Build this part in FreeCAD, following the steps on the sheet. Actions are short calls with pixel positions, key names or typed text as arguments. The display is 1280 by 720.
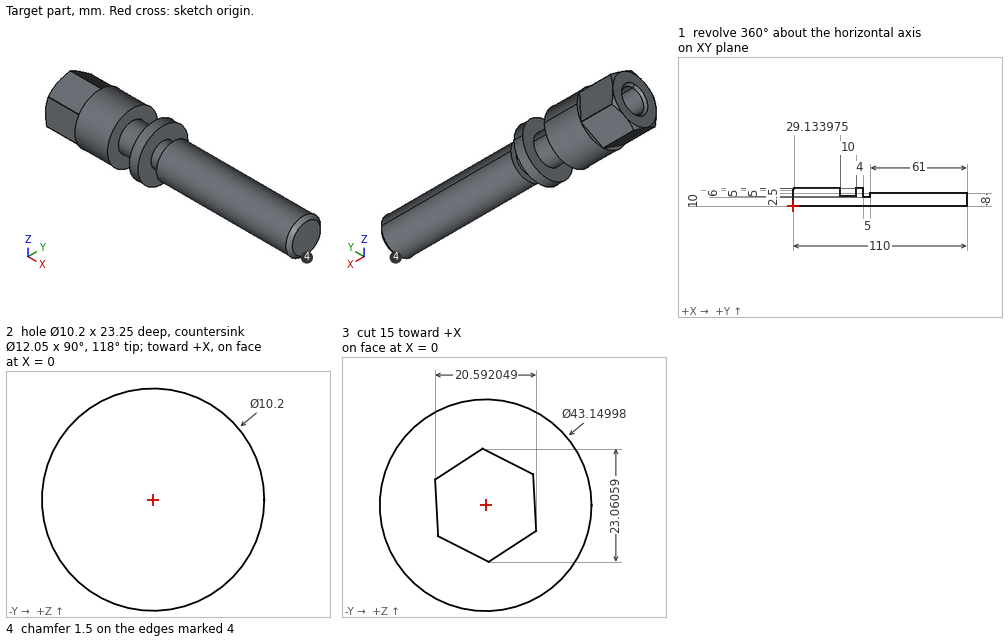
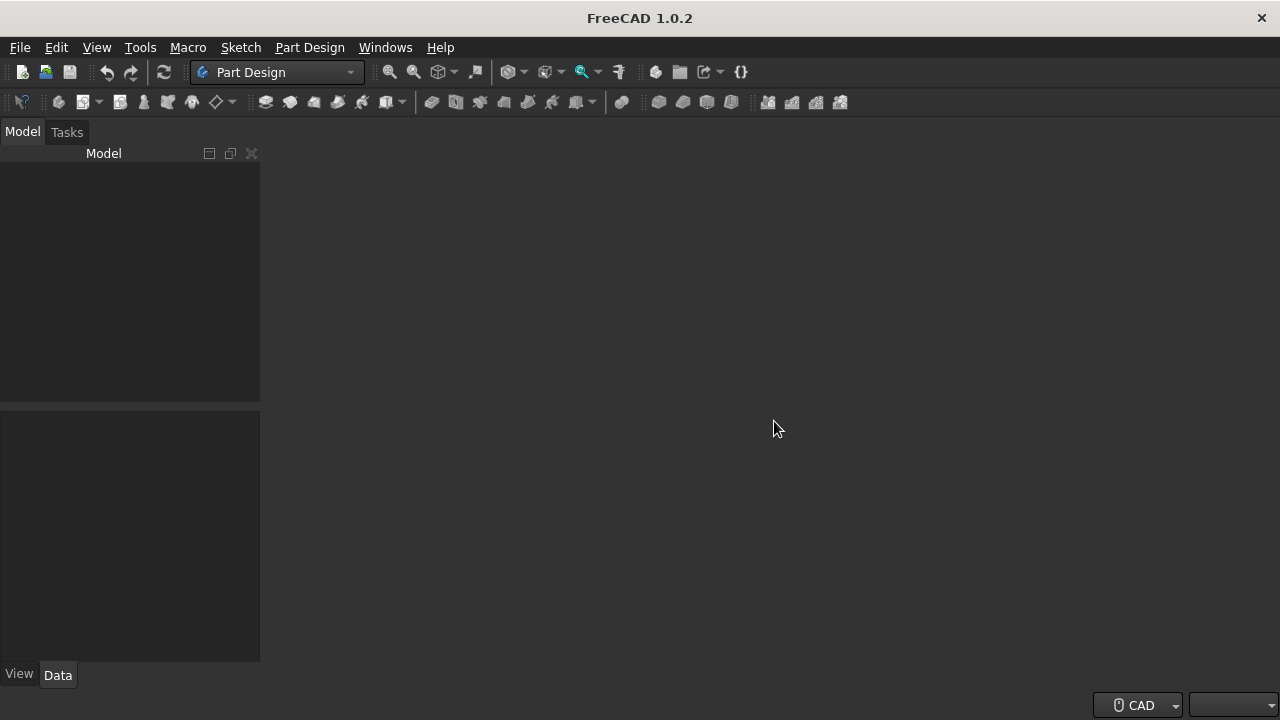
key(ctrl+n)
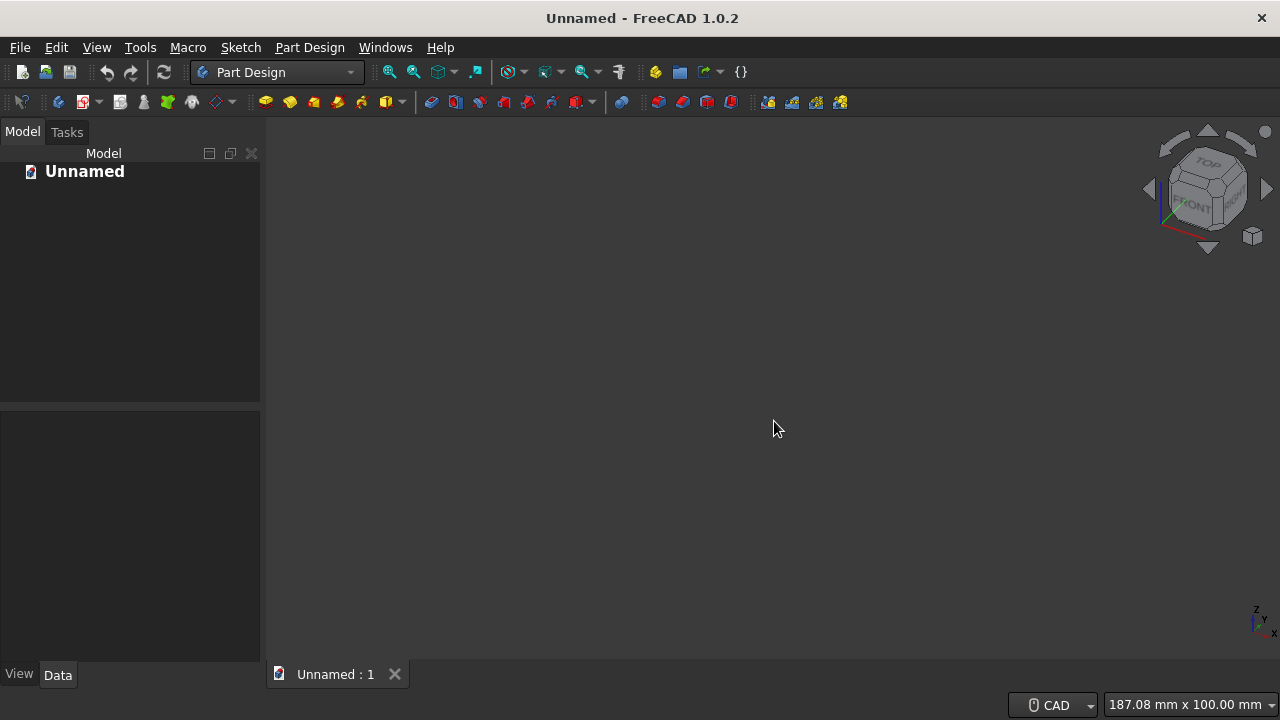
click(84, 102)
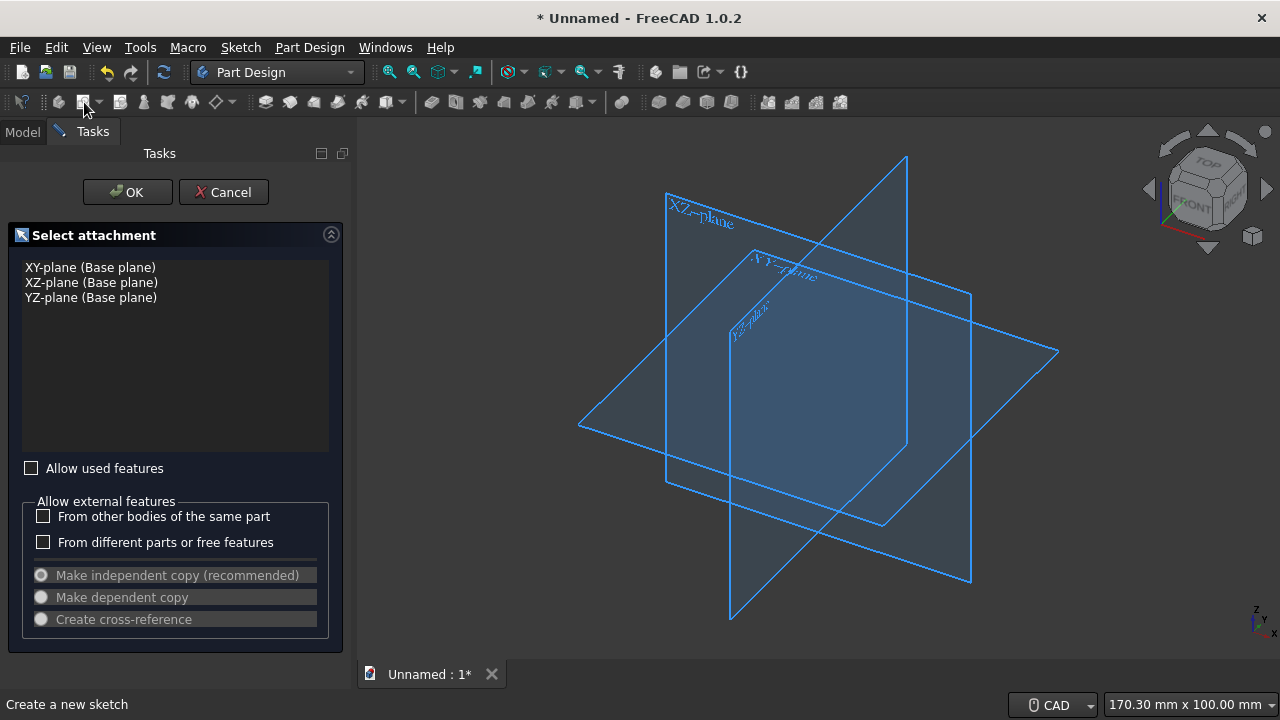
click(82, 268)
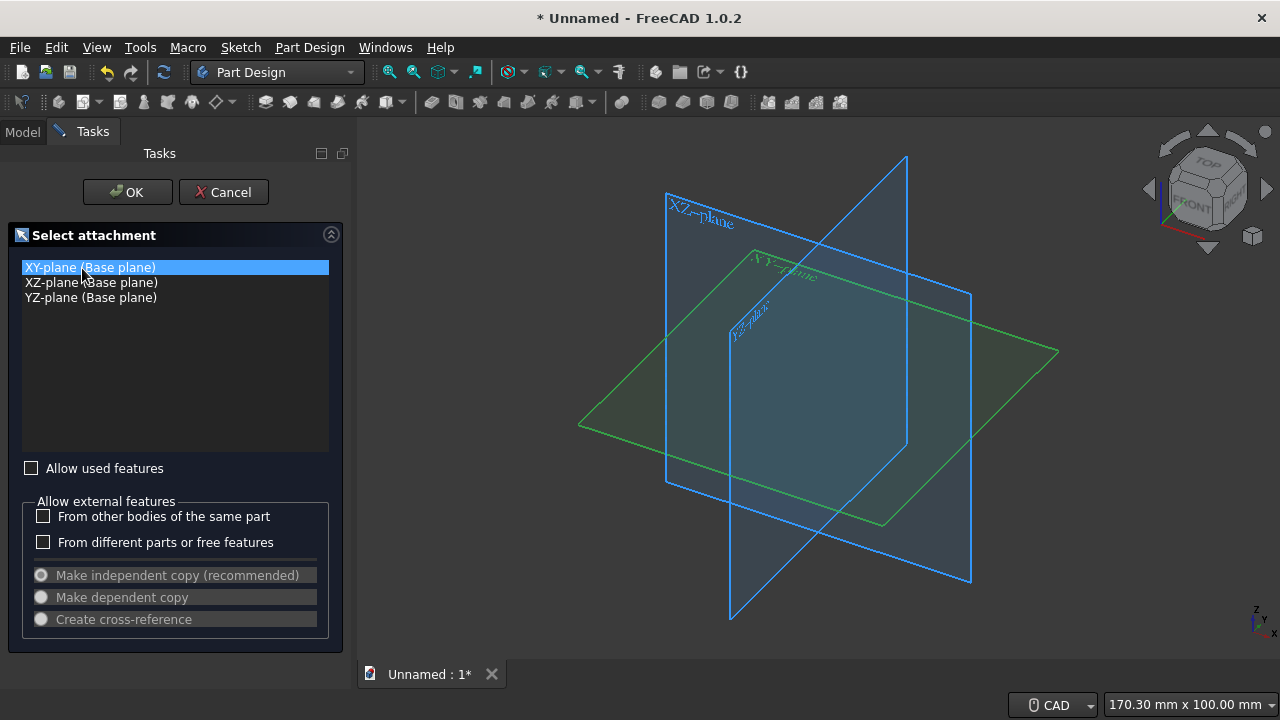
click(128, 192)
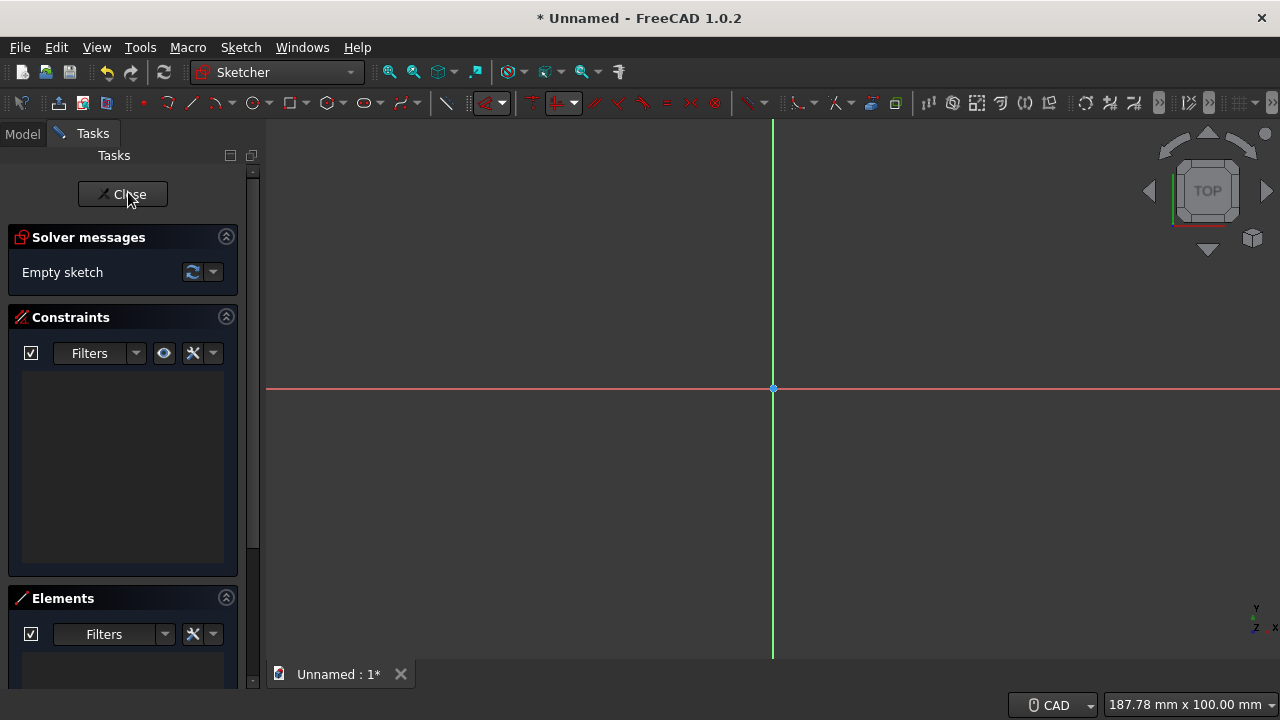
scroll(294, 452, down, 2)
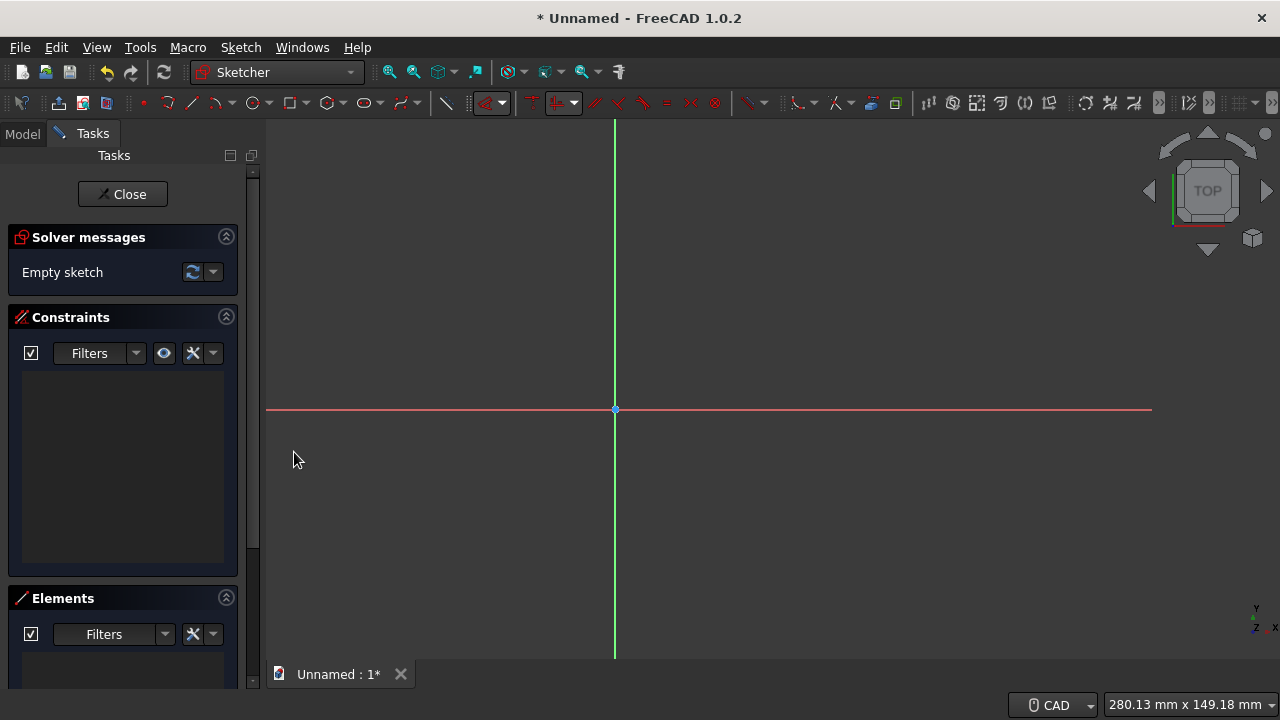
scroll(1037, 389, up, 2)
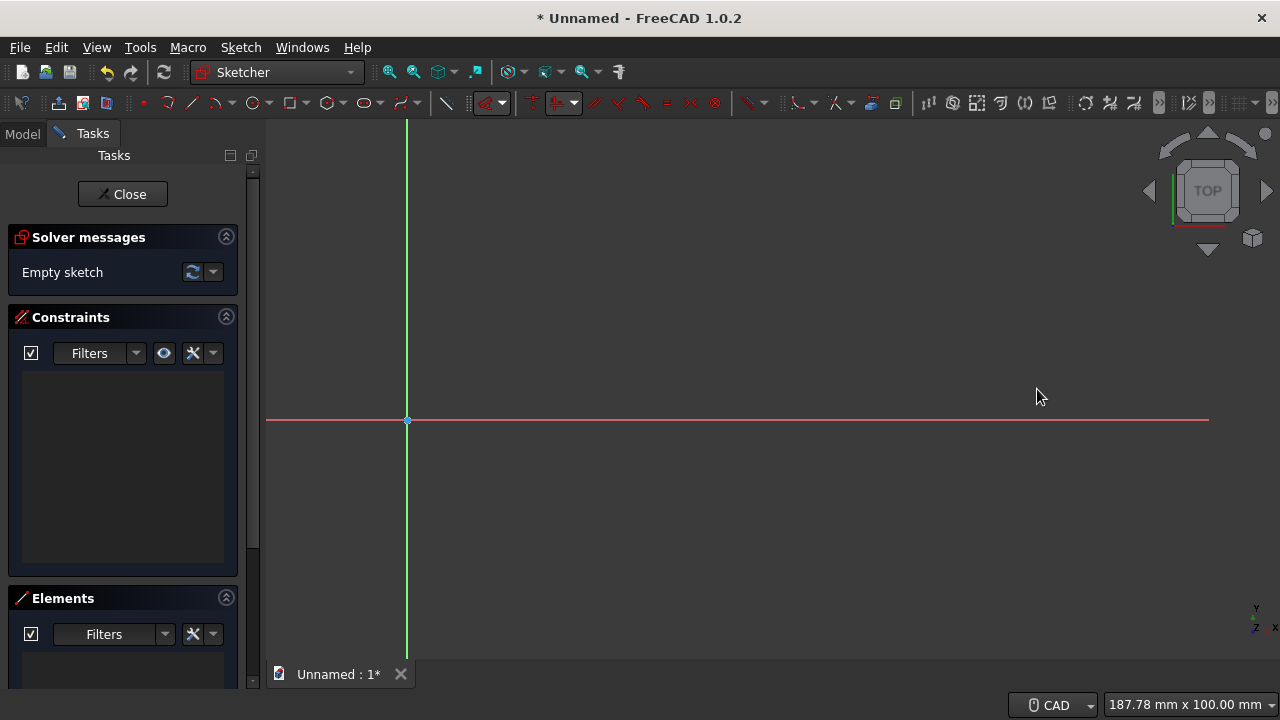
click(168, 104)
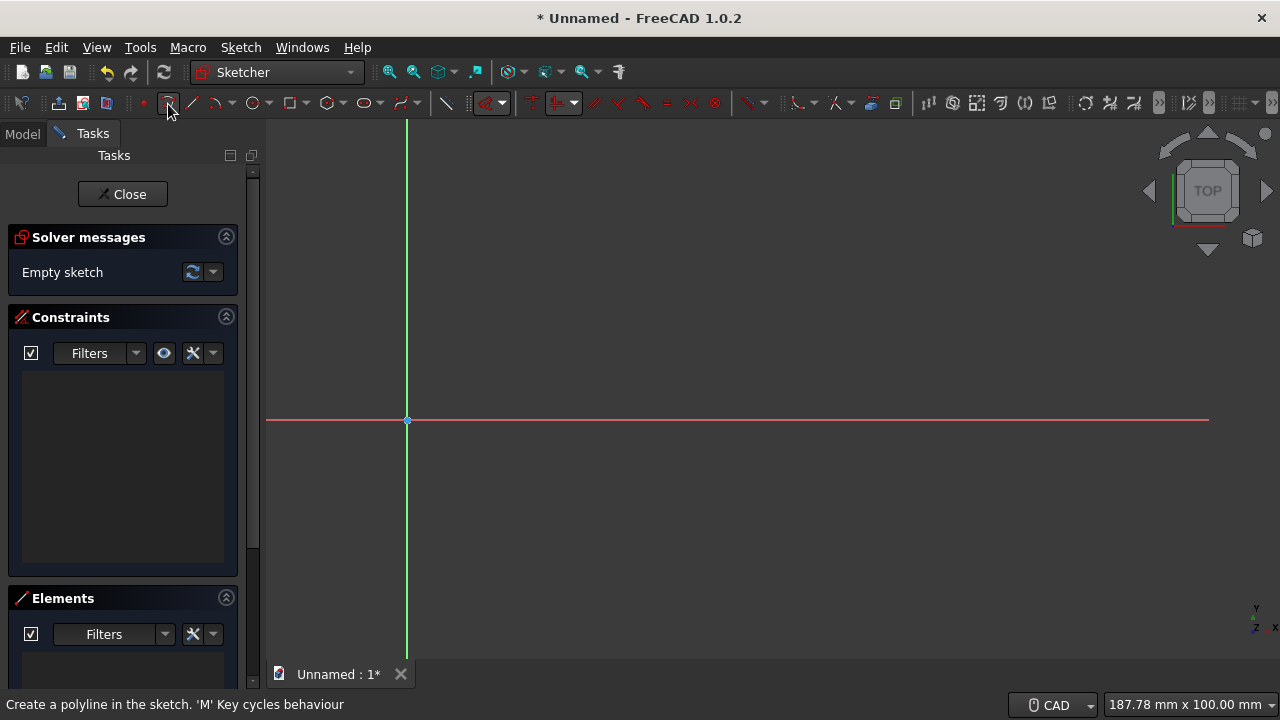
click(407, 420)
click(1001, 411)
click(1001, 377)
click(672, 377)
click(672, 390)
click(645, 390)
click(645, 358)
click(623, 358)
click(623, 385)
click(569, 385)
click(569, 358)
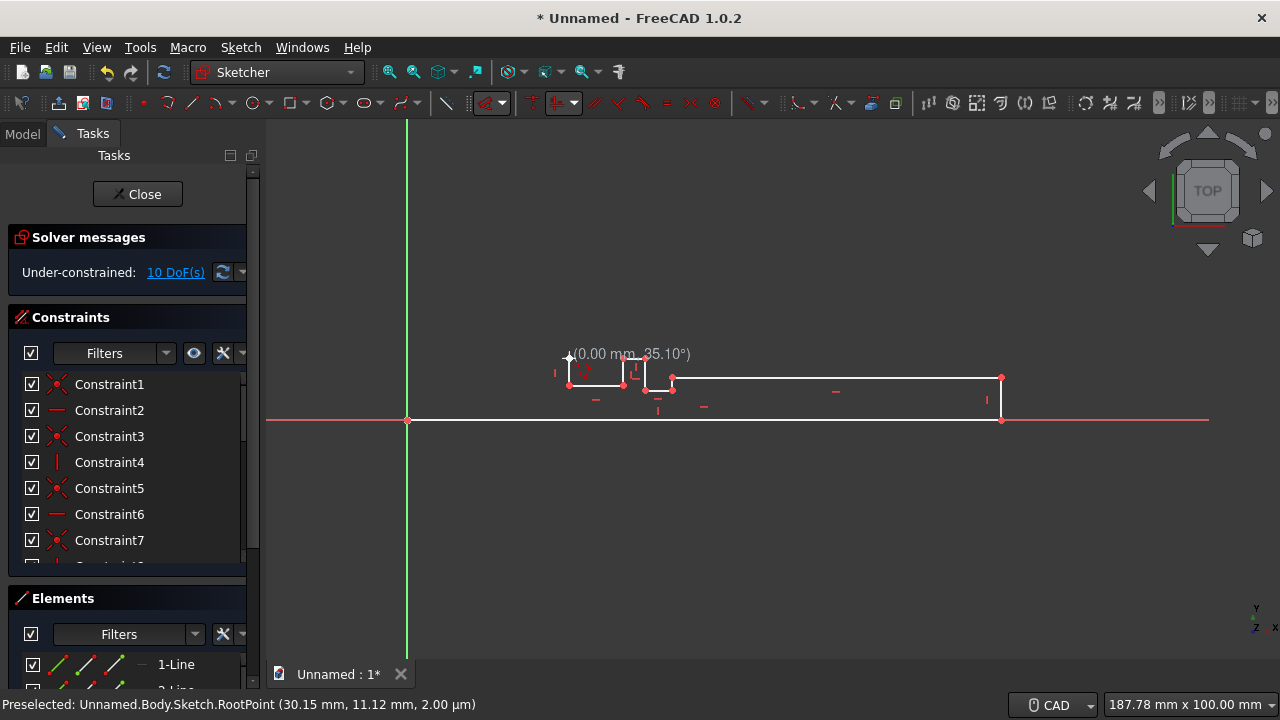
scroll(412, 358, up, 7)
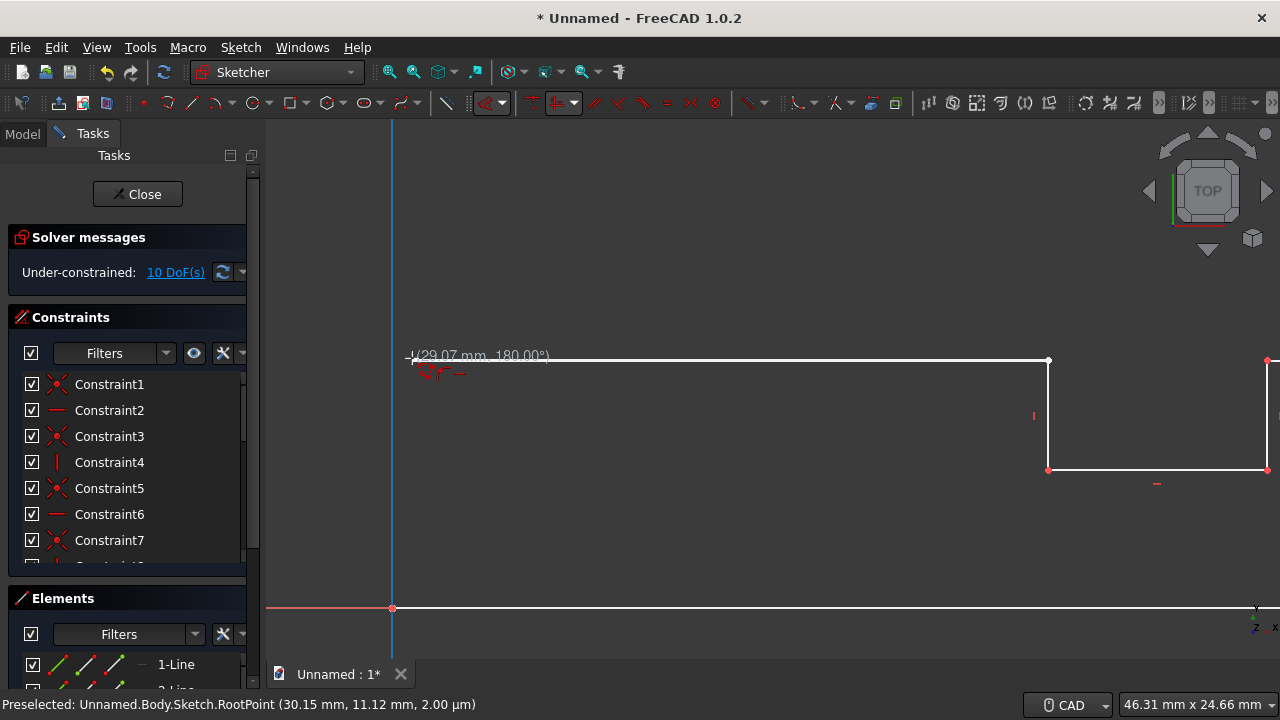
click(411, 357)
click(401, 389)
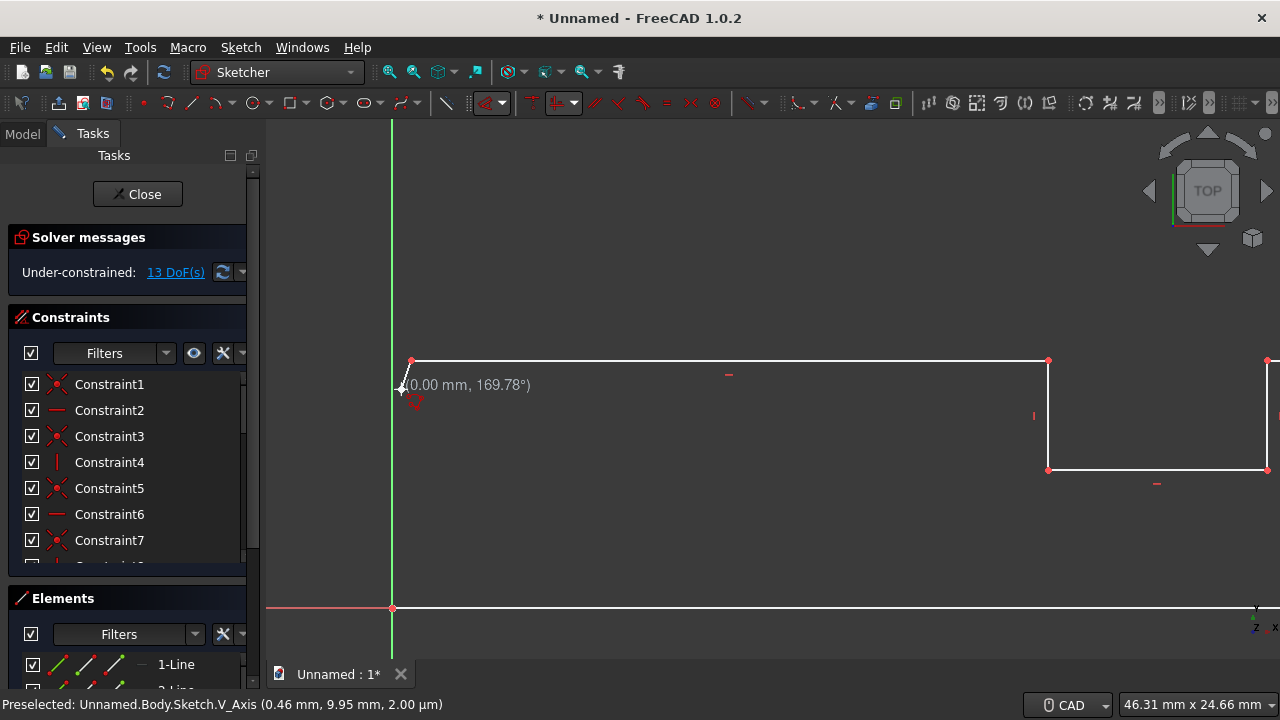
scroll(413, 358, down, 7)